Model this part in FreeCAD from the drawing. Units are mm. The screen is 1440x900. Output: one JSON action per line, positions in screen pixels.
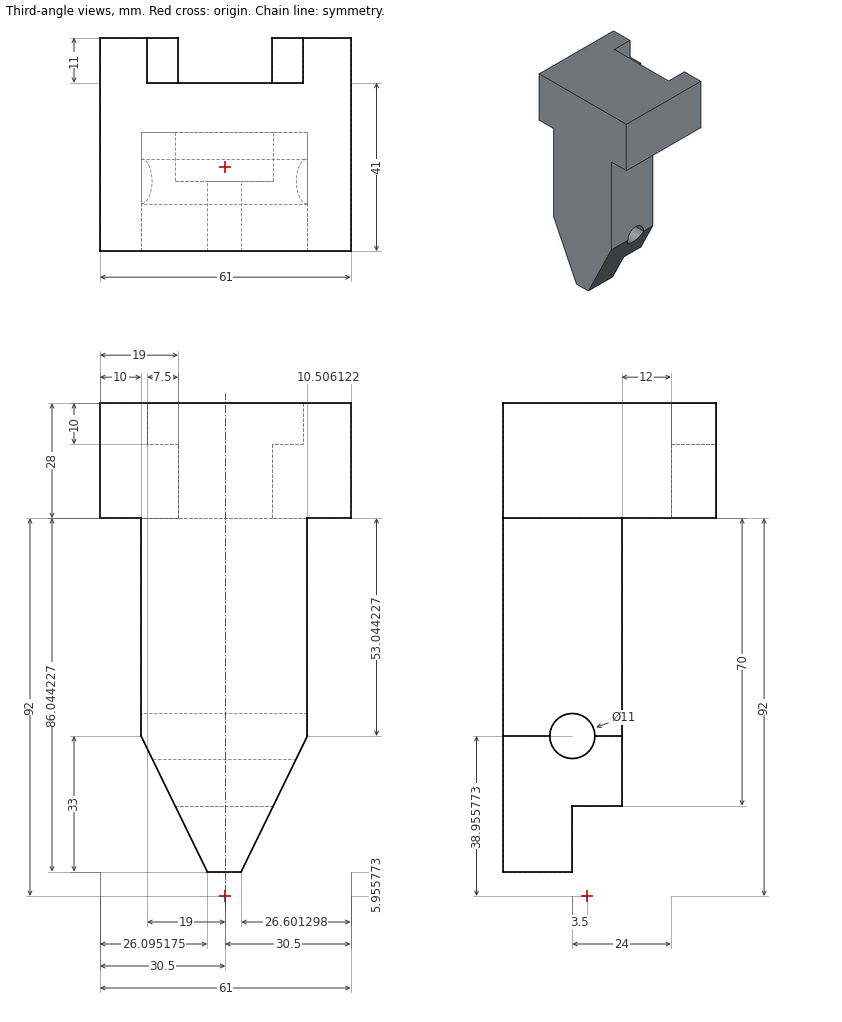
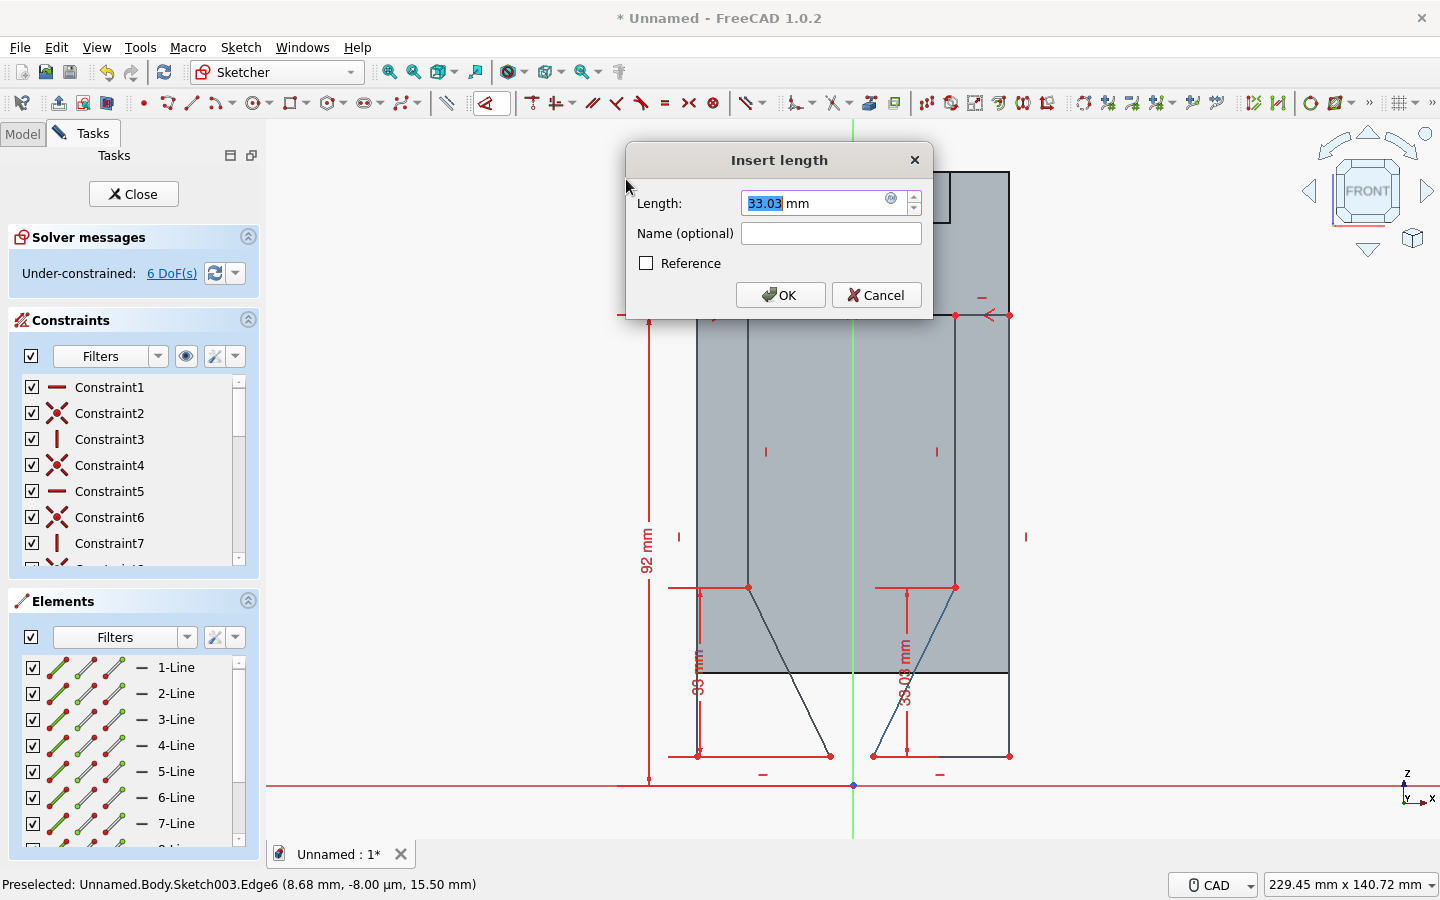
{"action": "type", "text": "33"}
{"action": "key", "text": "Return"}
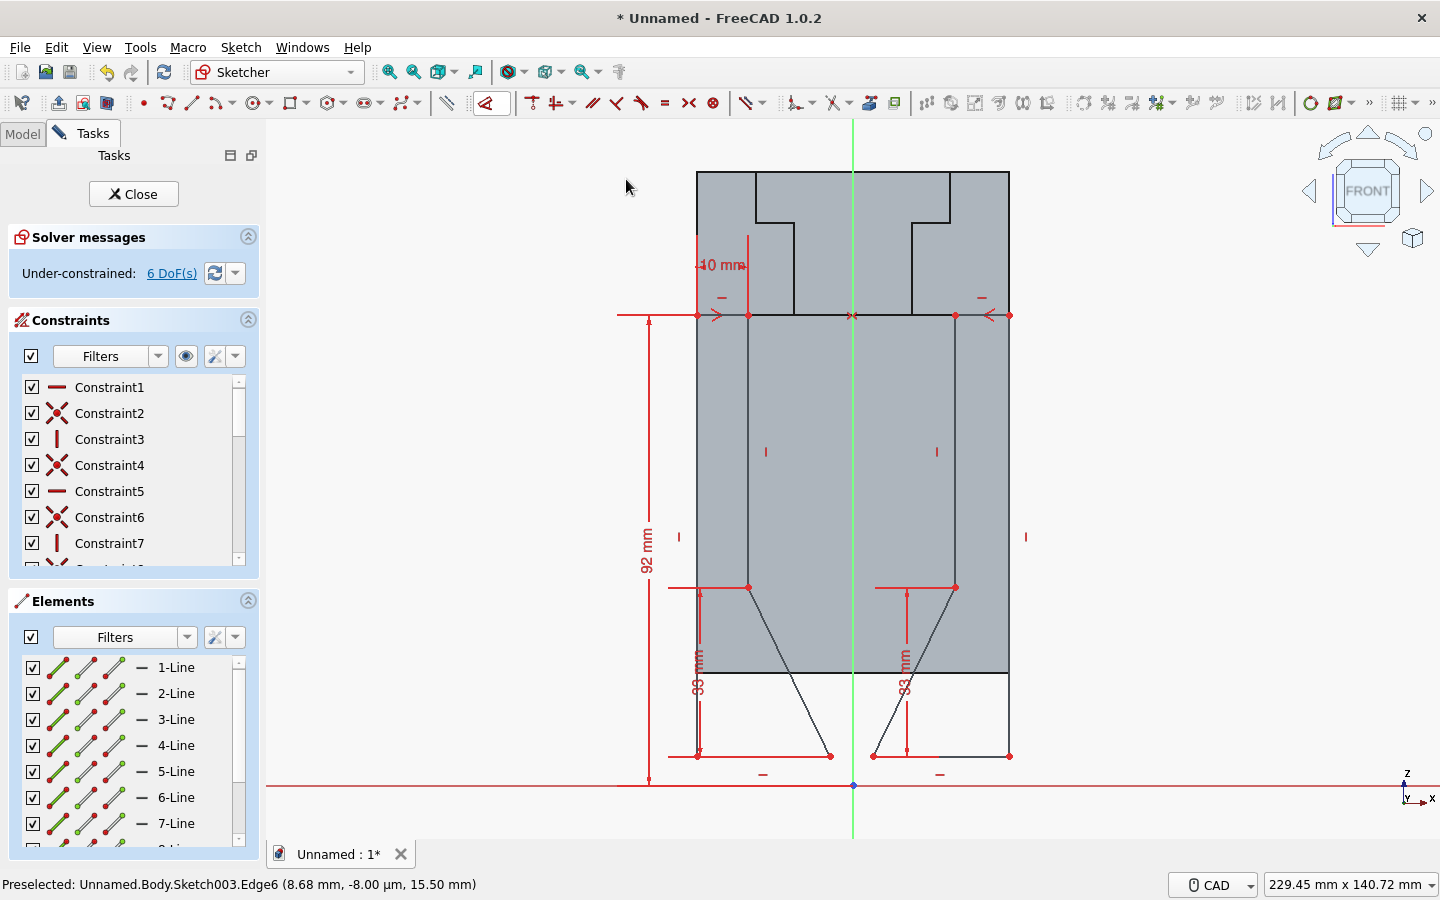
{"action": "left_click", "coordinate": [697, 757]}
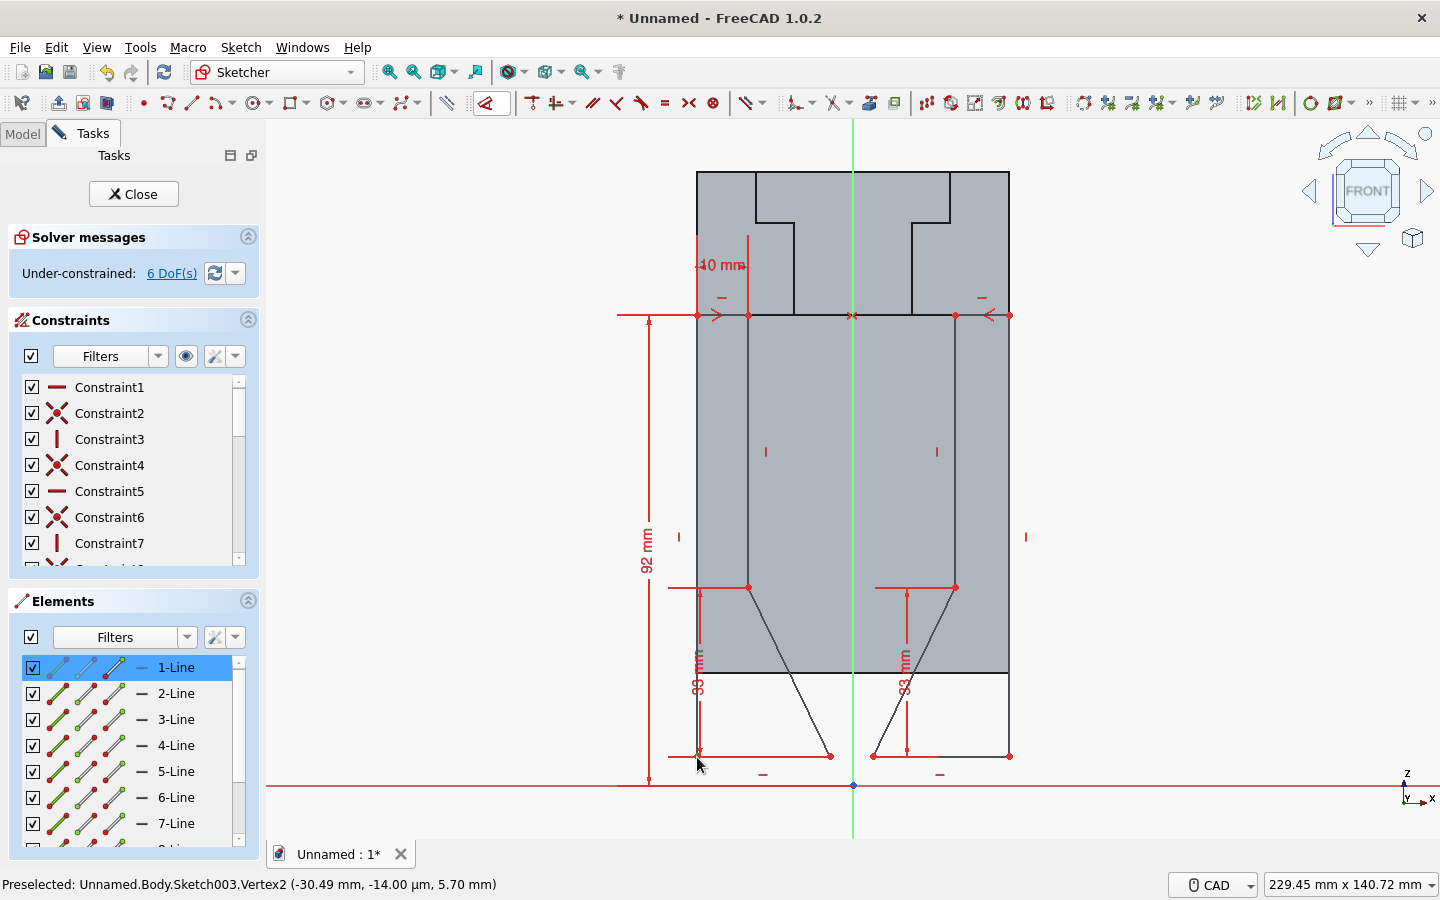
{"action": "key", "text": "l"}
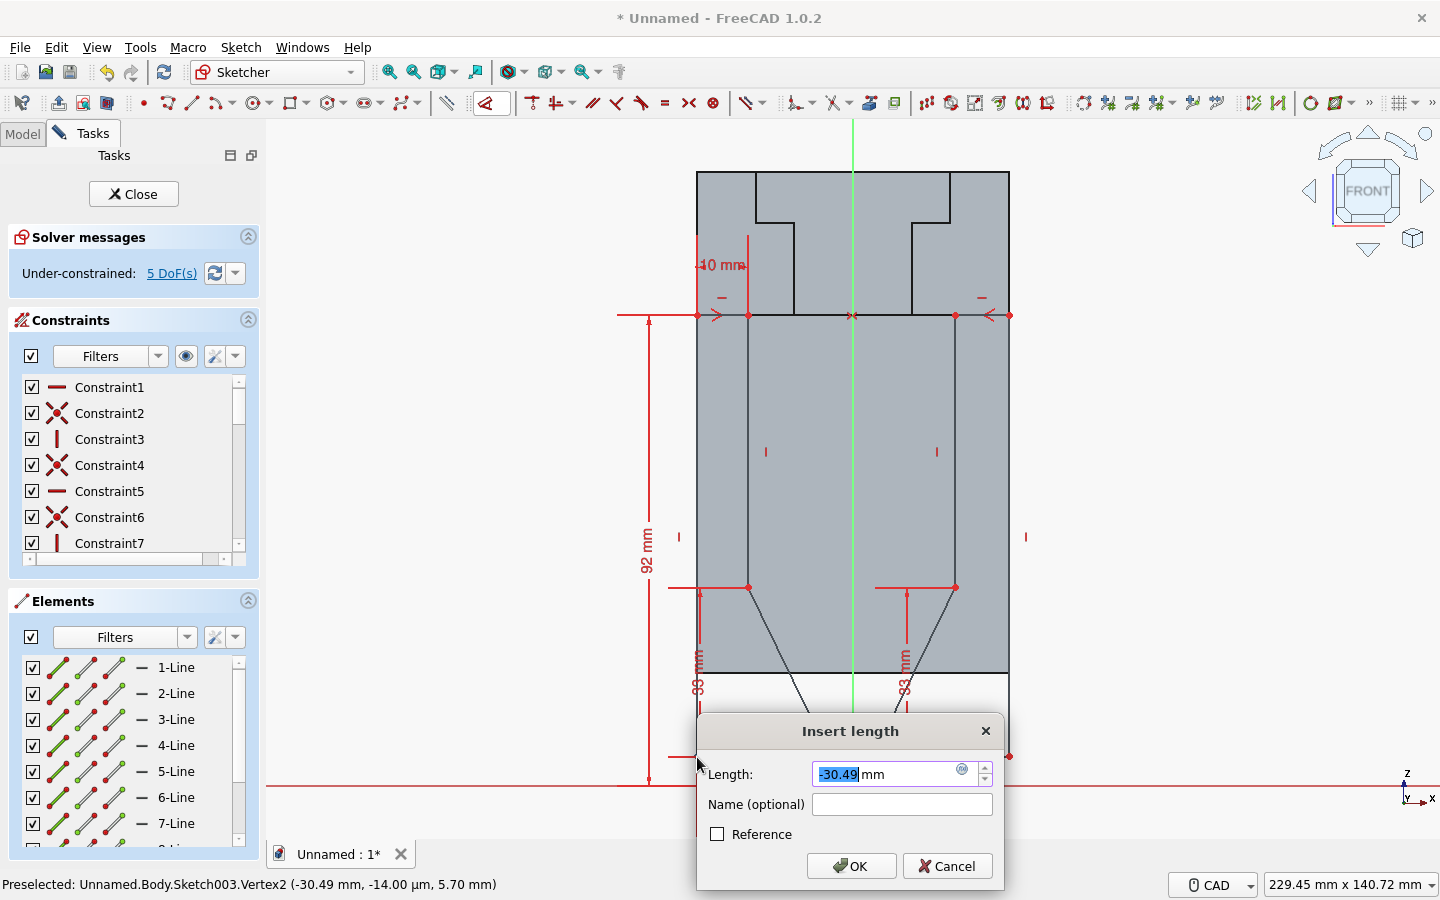
{"action": "type", "text": "-30.5"}
{"action": "key", "text": "Return"}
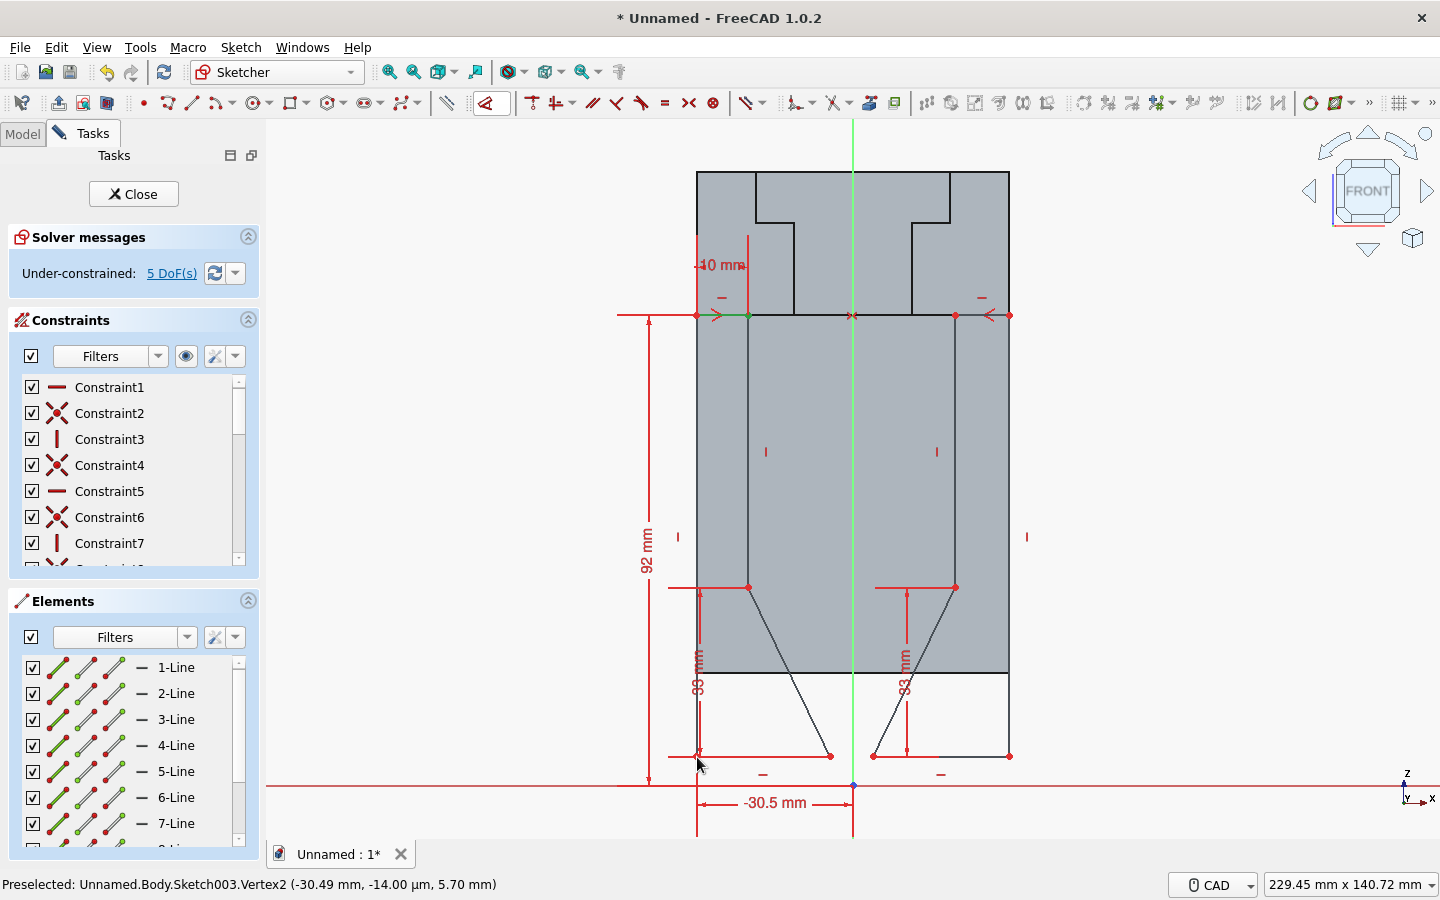
{"action": "left_click", "coordinate": [790, 757]}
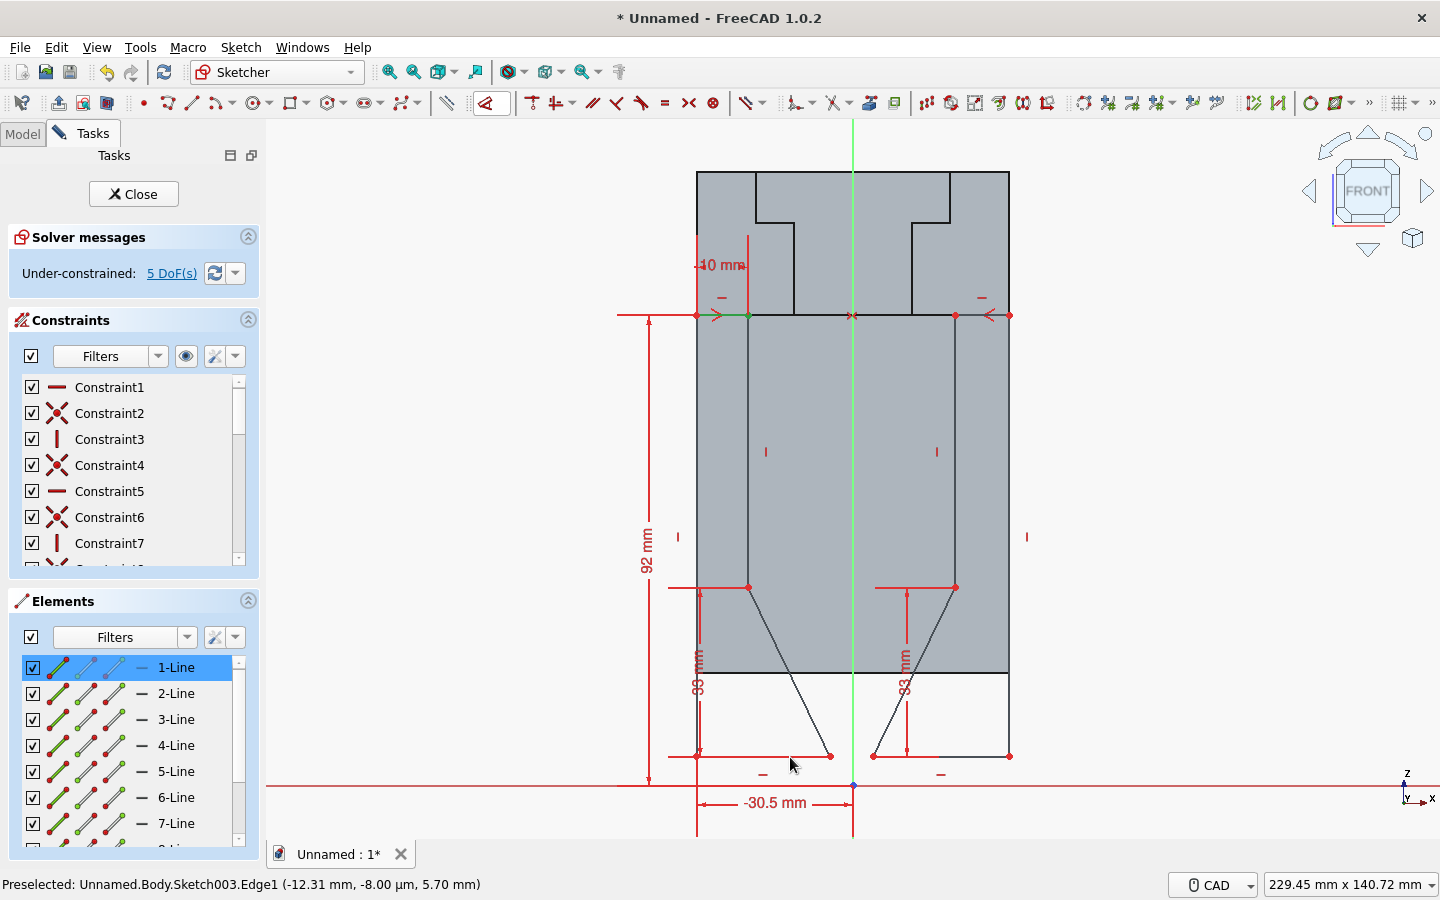
{"action": "left_click", "coordinate": [504, 104]}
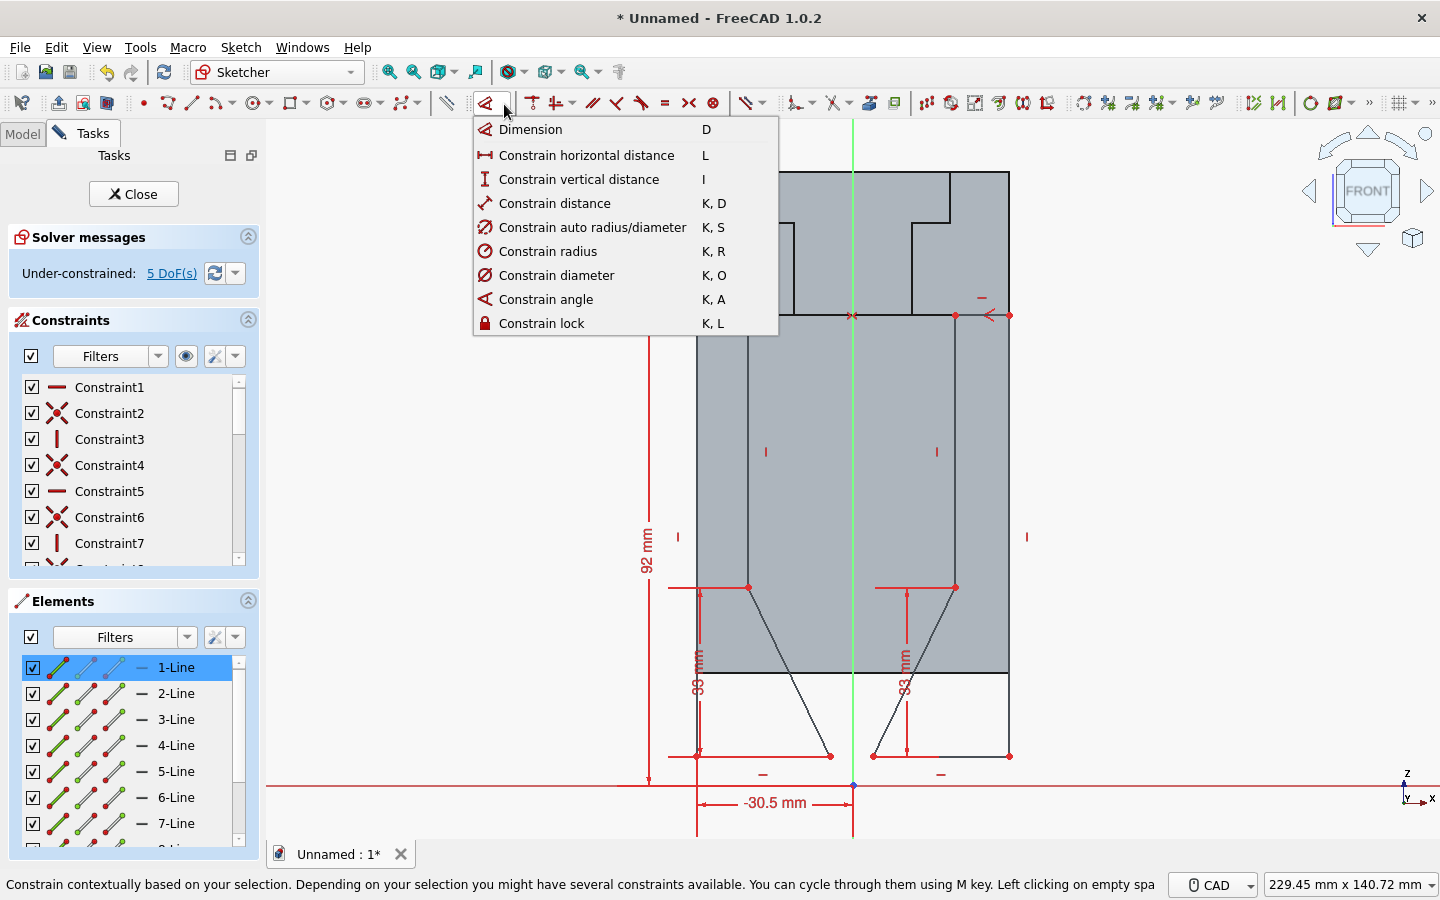
{"action": "left_click", "coordinate": [626, 155]}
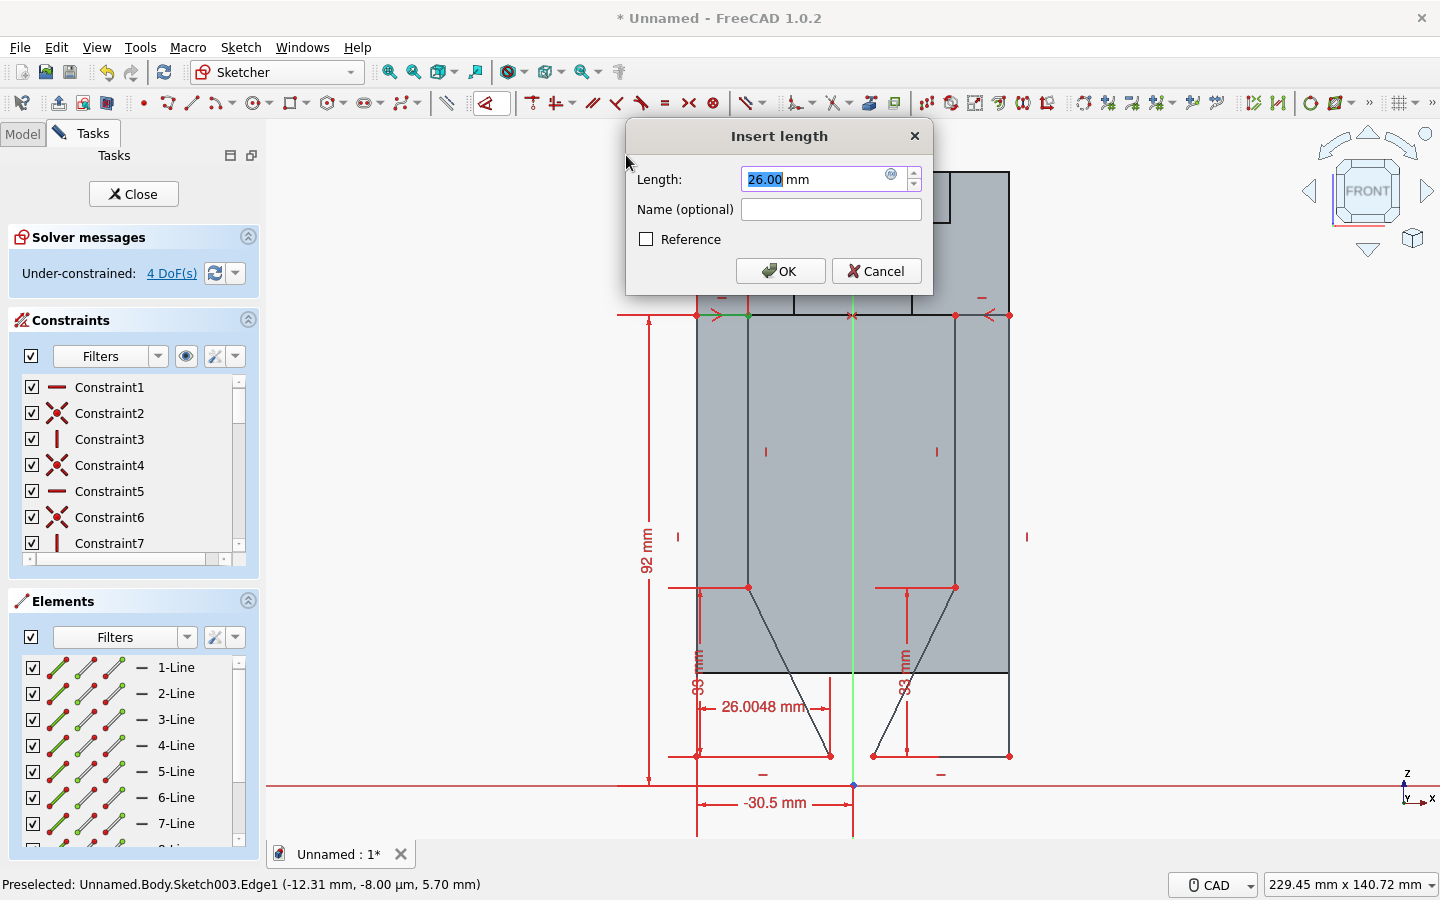
{"action": "type", "text": "26.095175"}
{"action": "key", "text": "Return"}